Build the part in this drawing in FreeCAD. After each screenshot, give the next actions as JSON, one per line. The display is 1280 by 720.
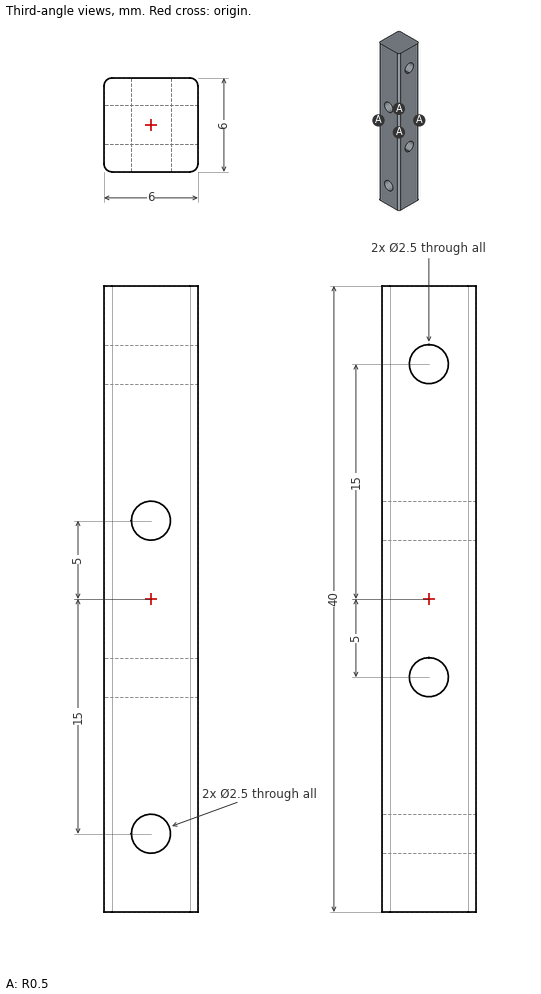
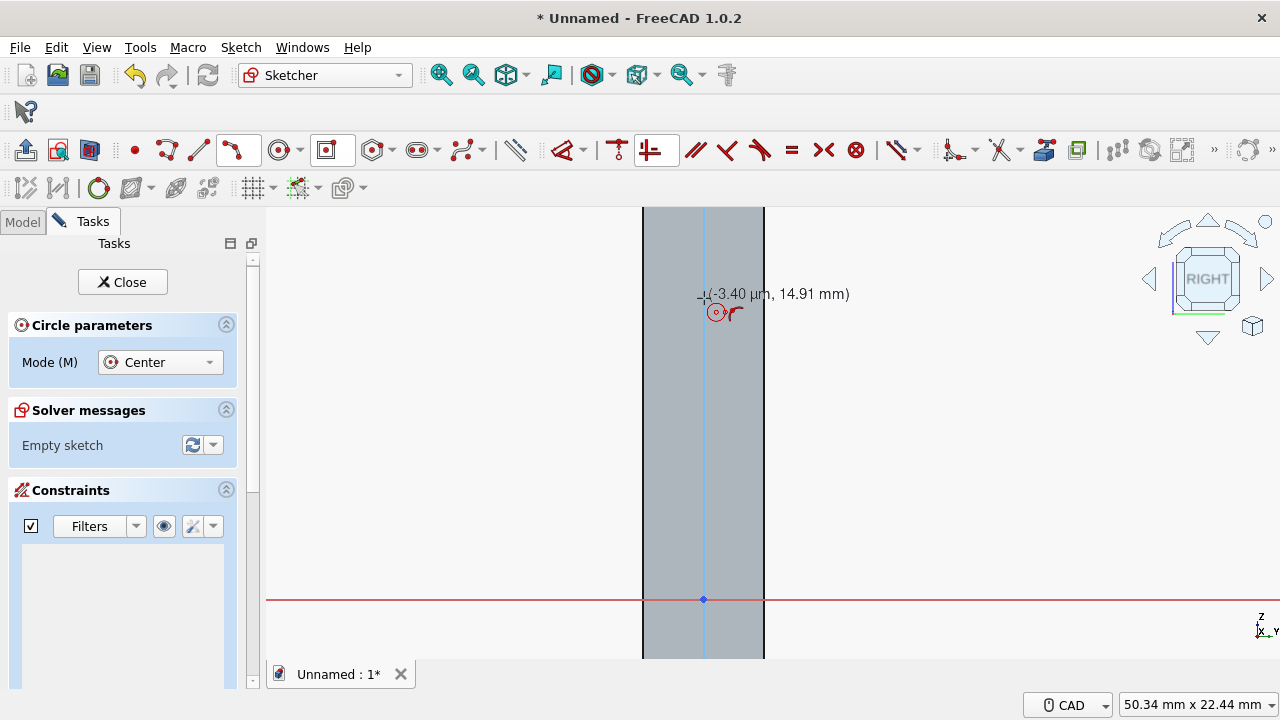
{"action": "left_click", "coordinate": [704, 298]}
{"action": "left_click", "coordinate": [722, 280]}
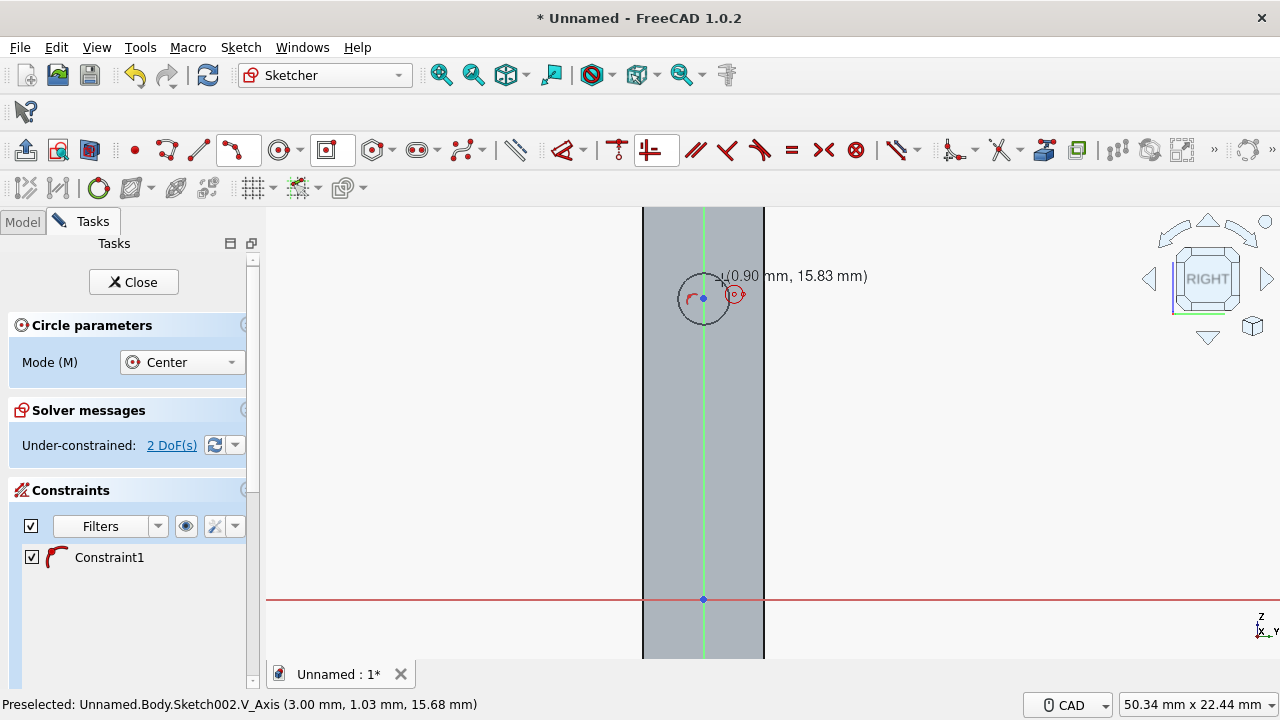
{"action": "scroll", "coordinate": [706, 299], "scroll_direction": "down", "scroll_amount": 2}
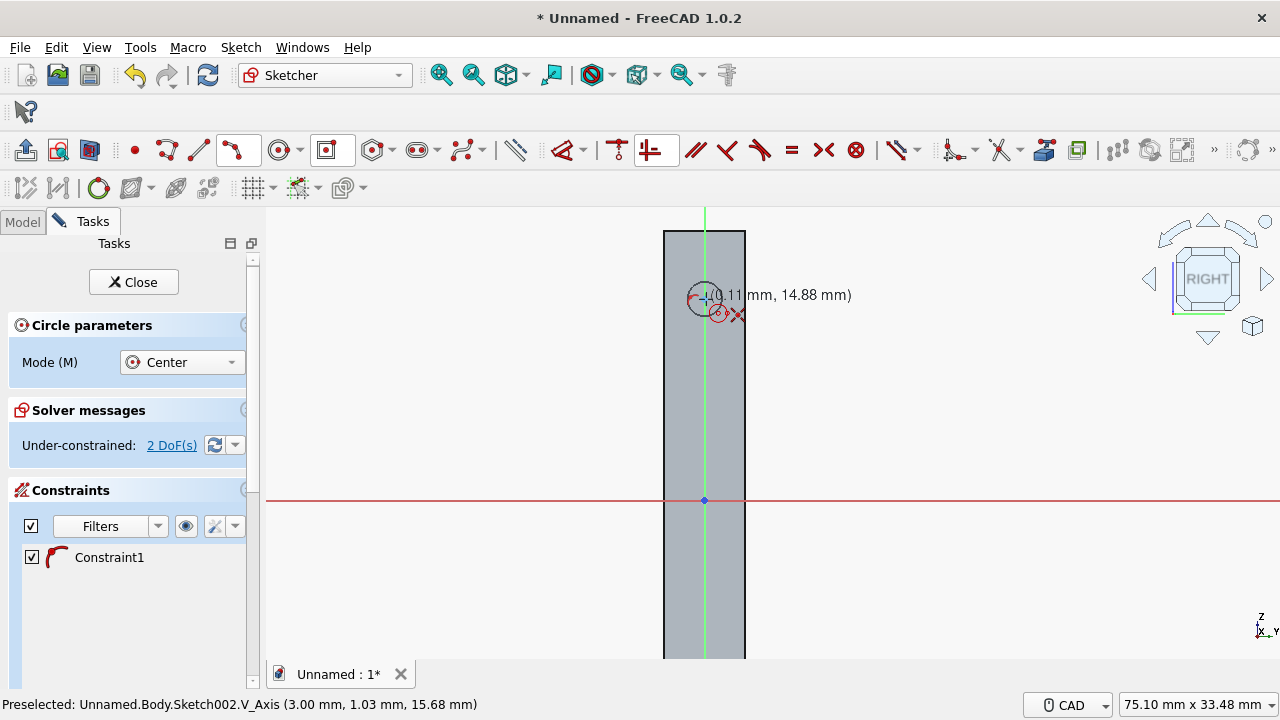
{"action": "scroll", "coordinate": [705, 568], "scroll_direction": "up", "scroll_amount": 2}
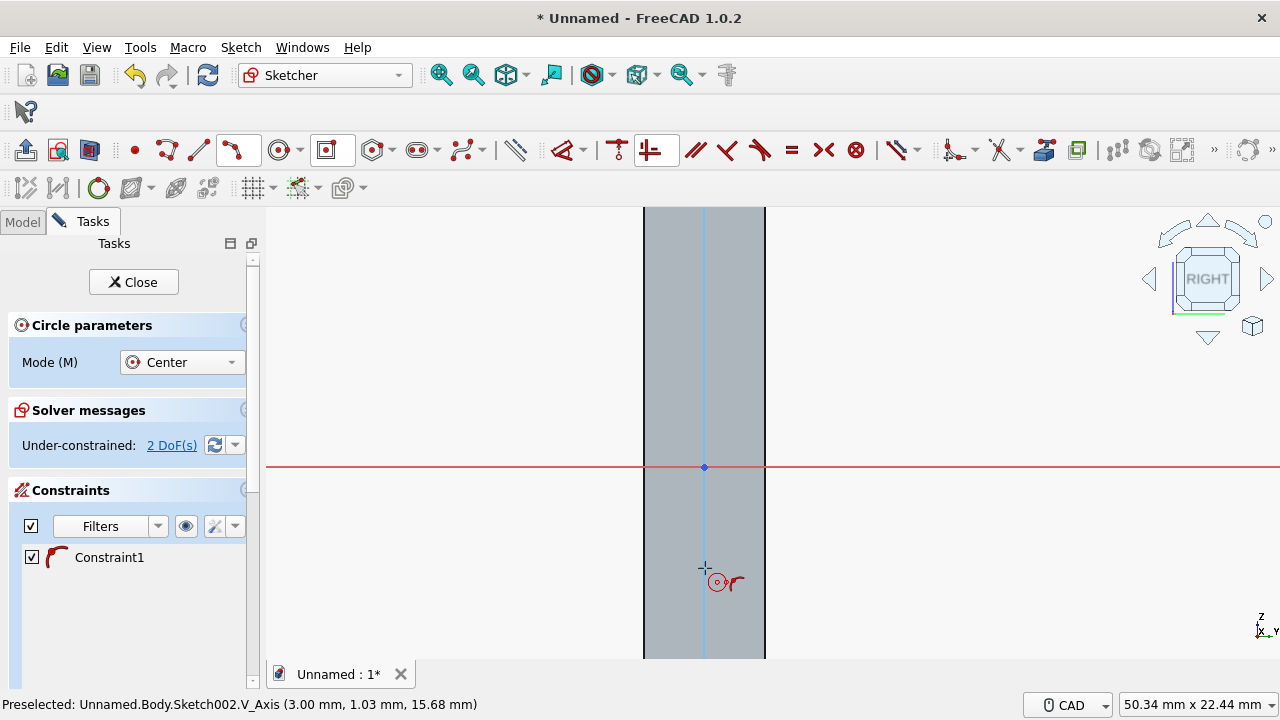
{"action": "left_click", "coordinate": [704, 568]}
{"action": "left_click", "coordinate": [722, 550]}
{"action": "key", "text": "Escape"}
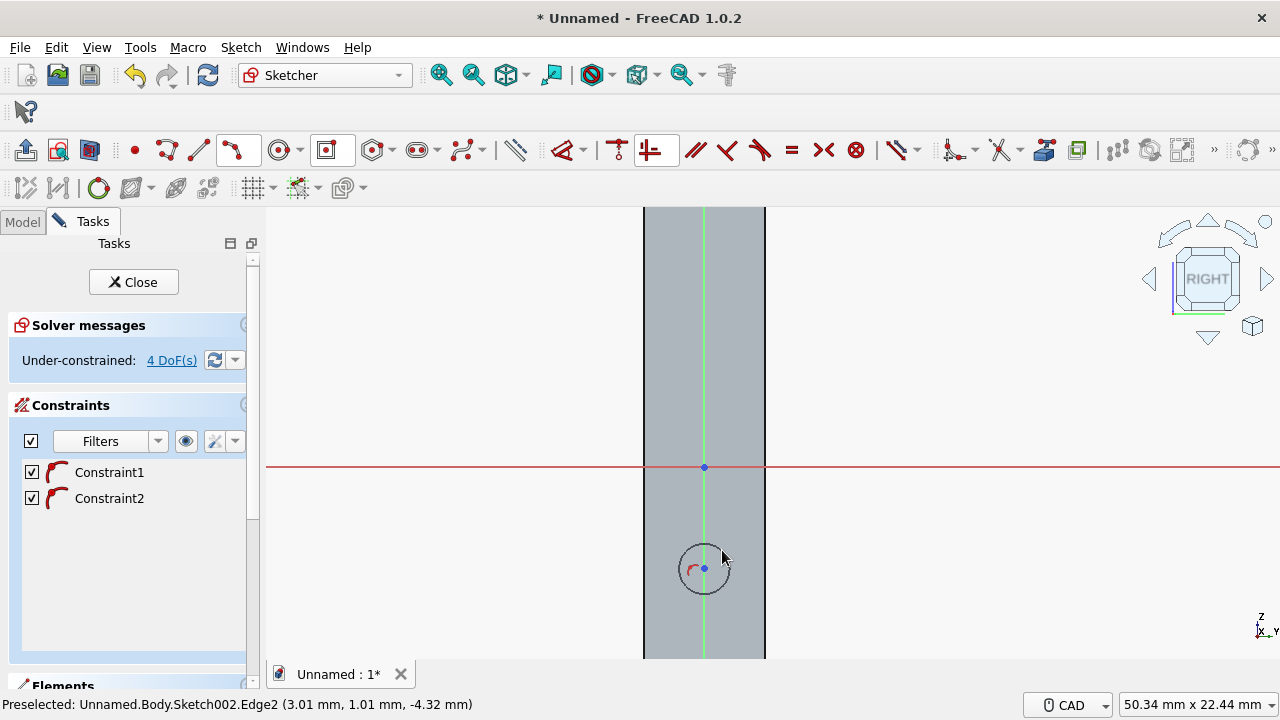
{"action": "scroll", "coordinate": [705, 568], "scroll_direction": "down", "scroll_amount": 2}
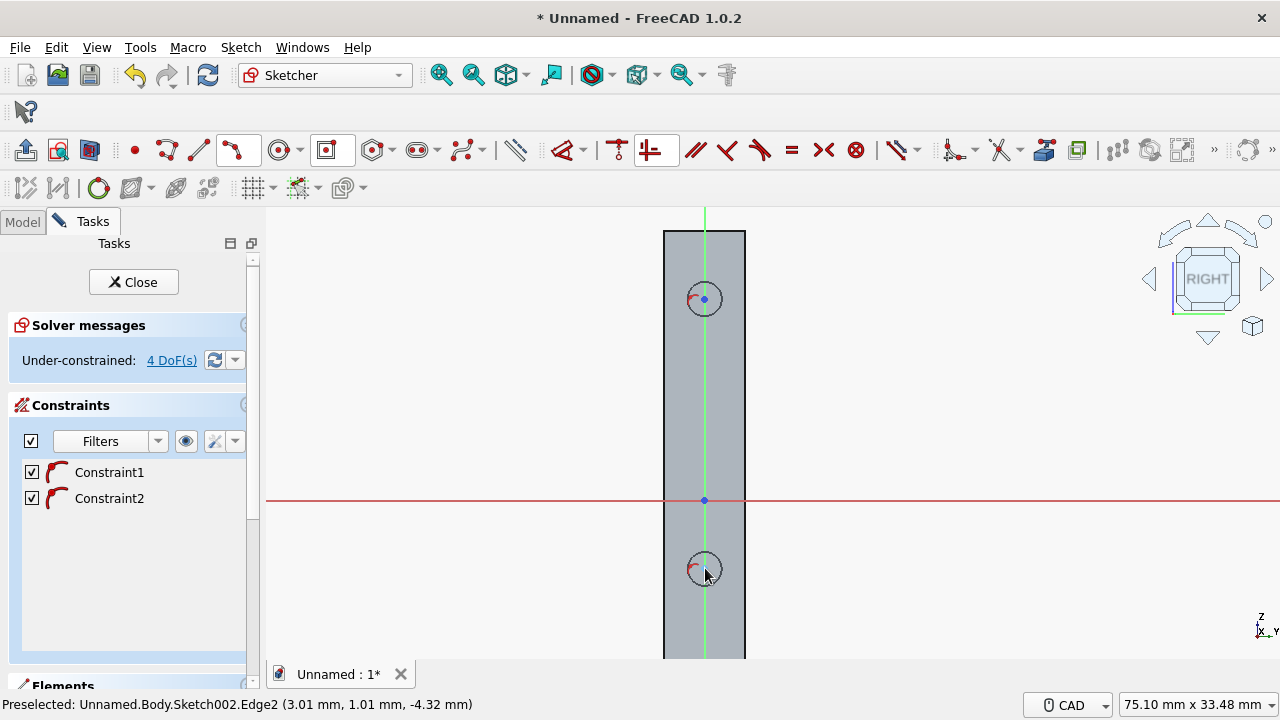
{"action": "left_click", "coordinate": [717, 287]}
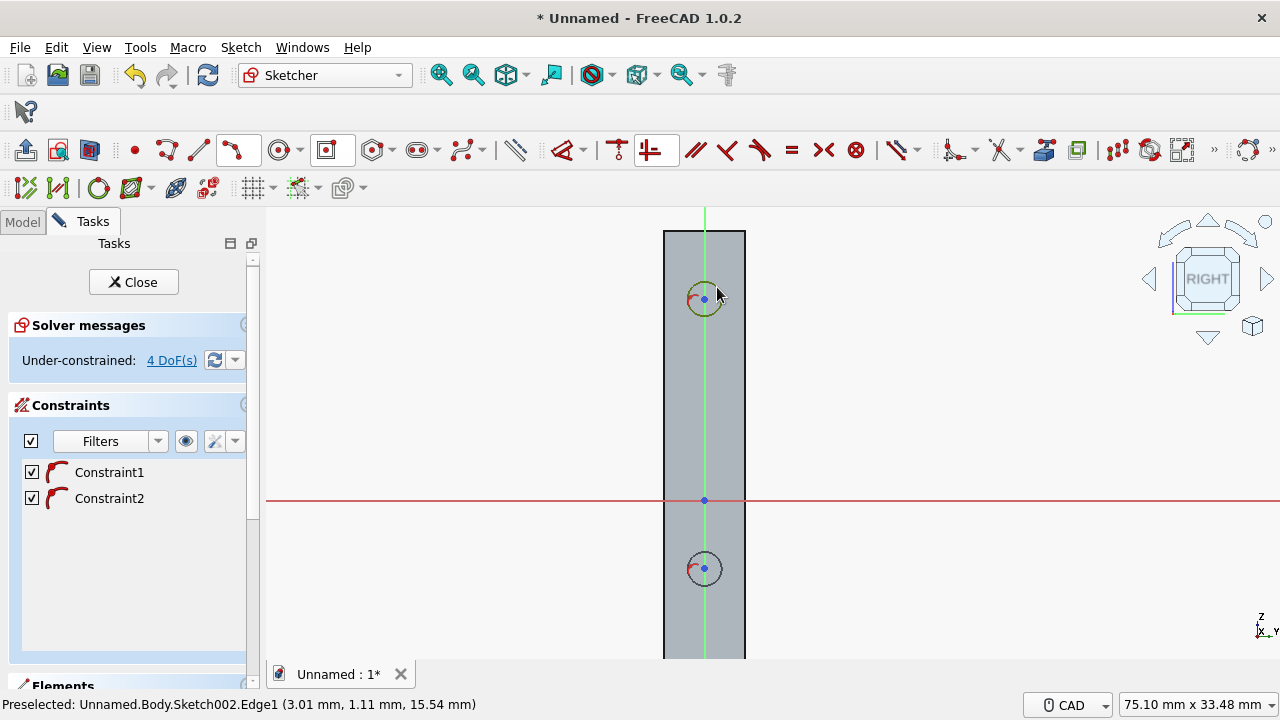
{"action": "left_click", "coordinate": [717, 557]}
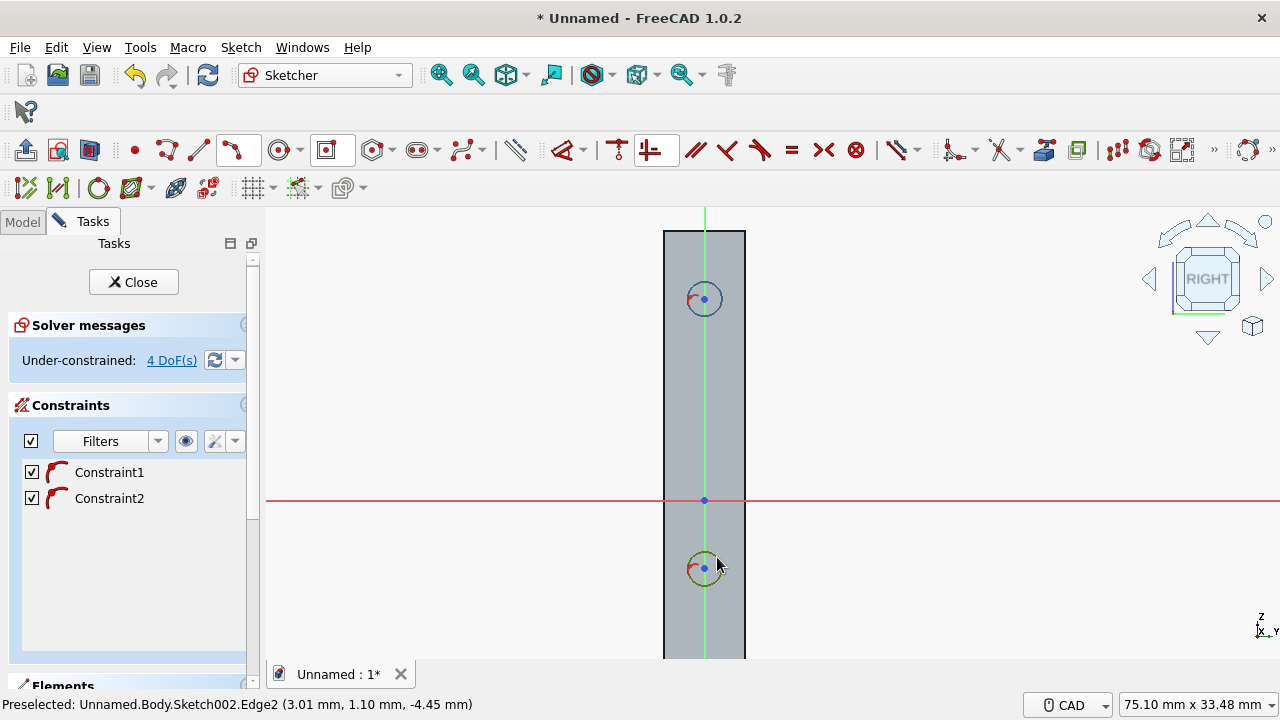
{"action": "left_click", "coordinate": [792, 150]}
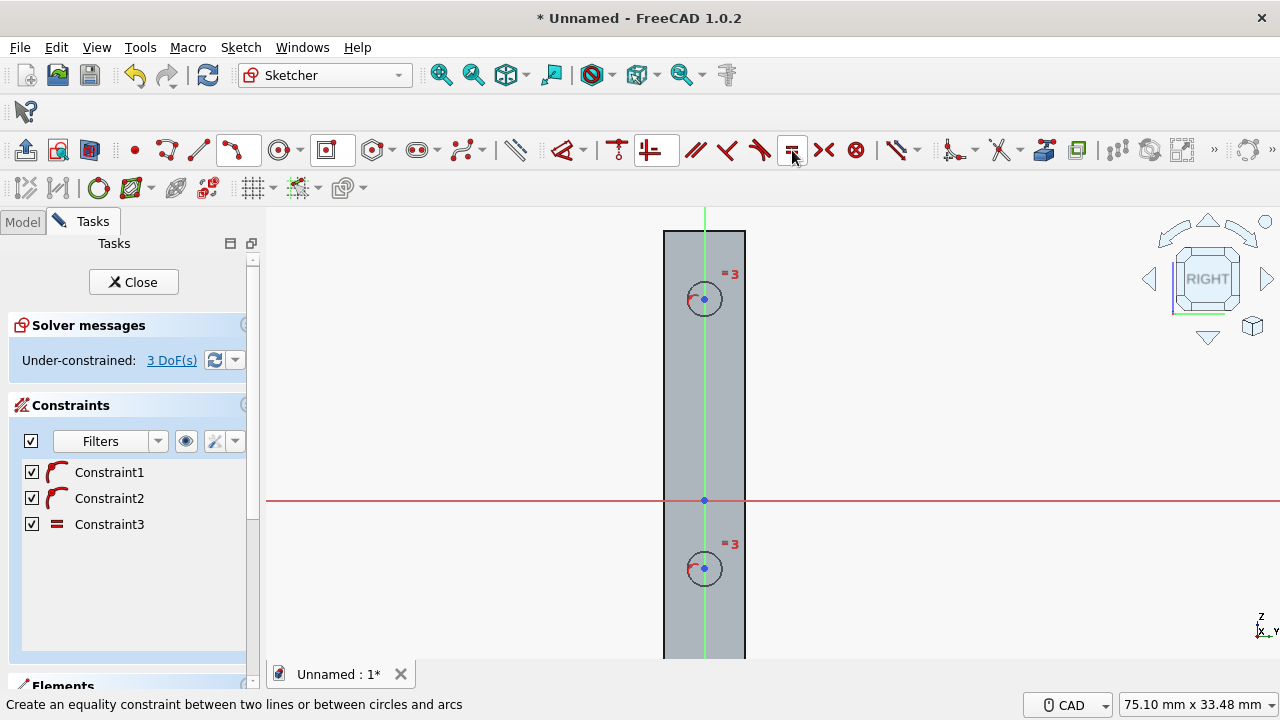
{"action": "left_click", "coordinate": [562, 150]}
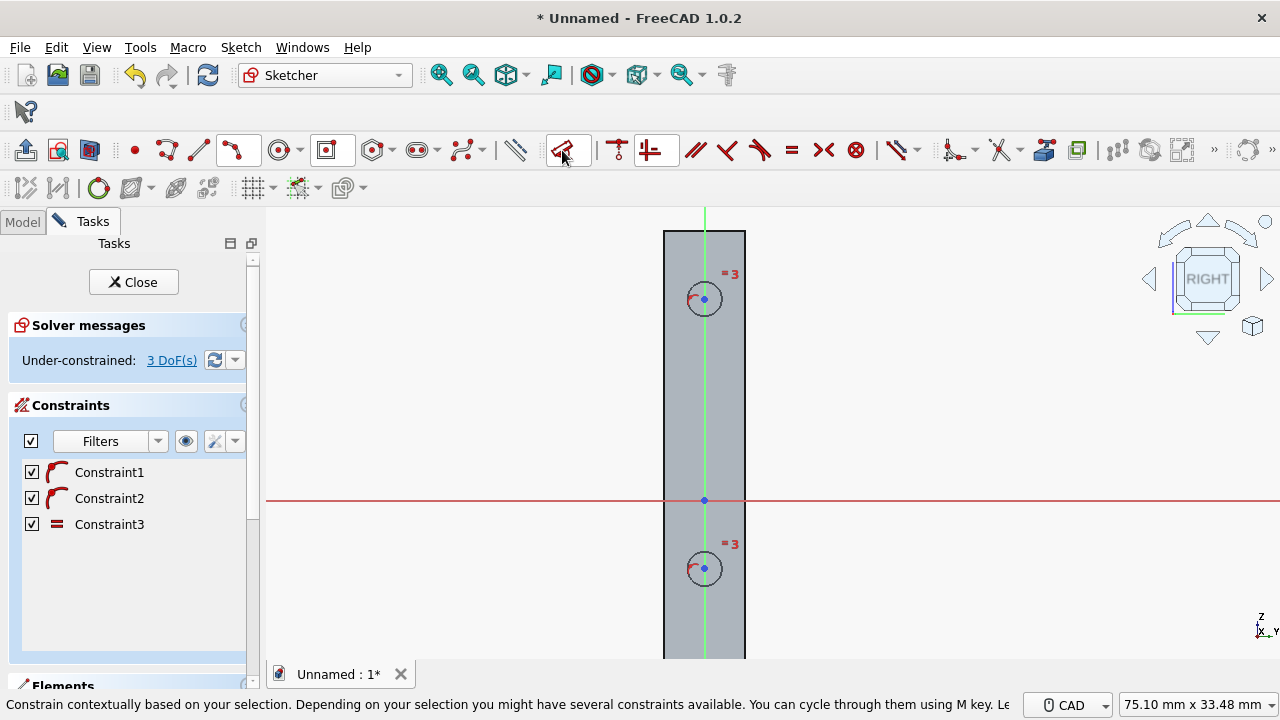
{"action": "left_click", "coordinate": [717, 287]}
{"action": "left_click", "coordinate": [740, 265]}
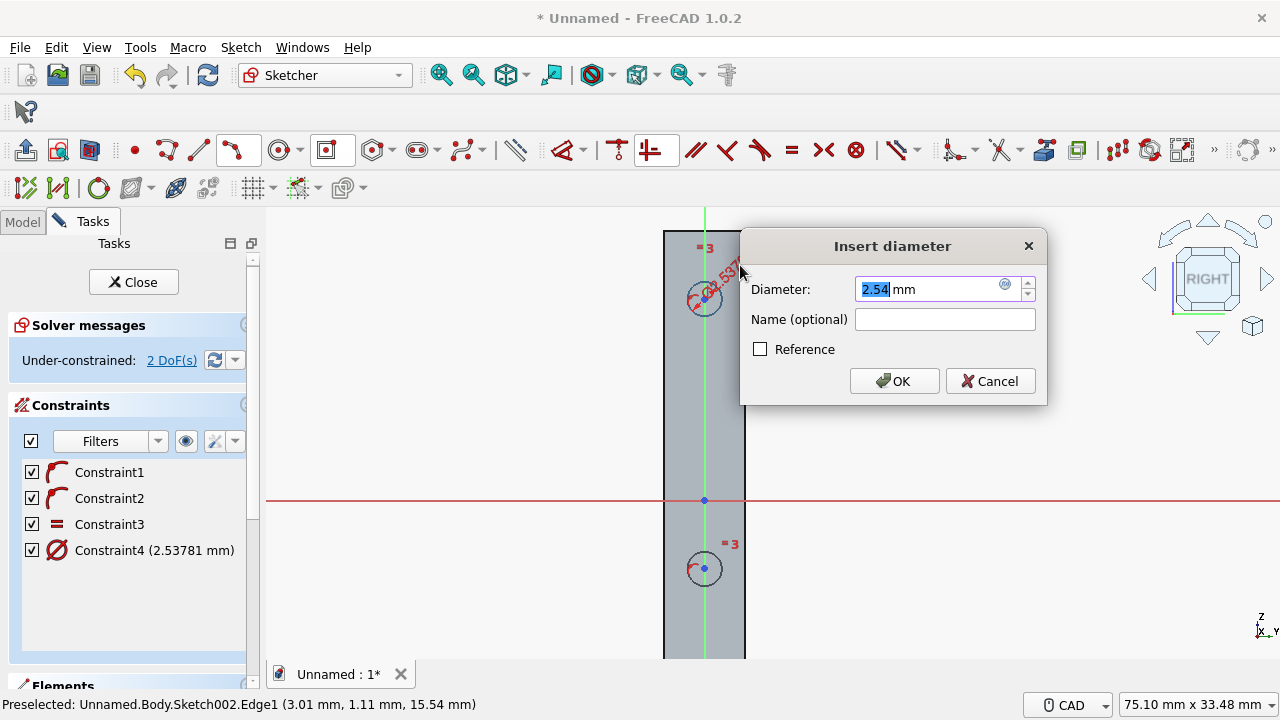
{"action": "type", "text": "2.5"}
{"action": "key", "text": "Return"}